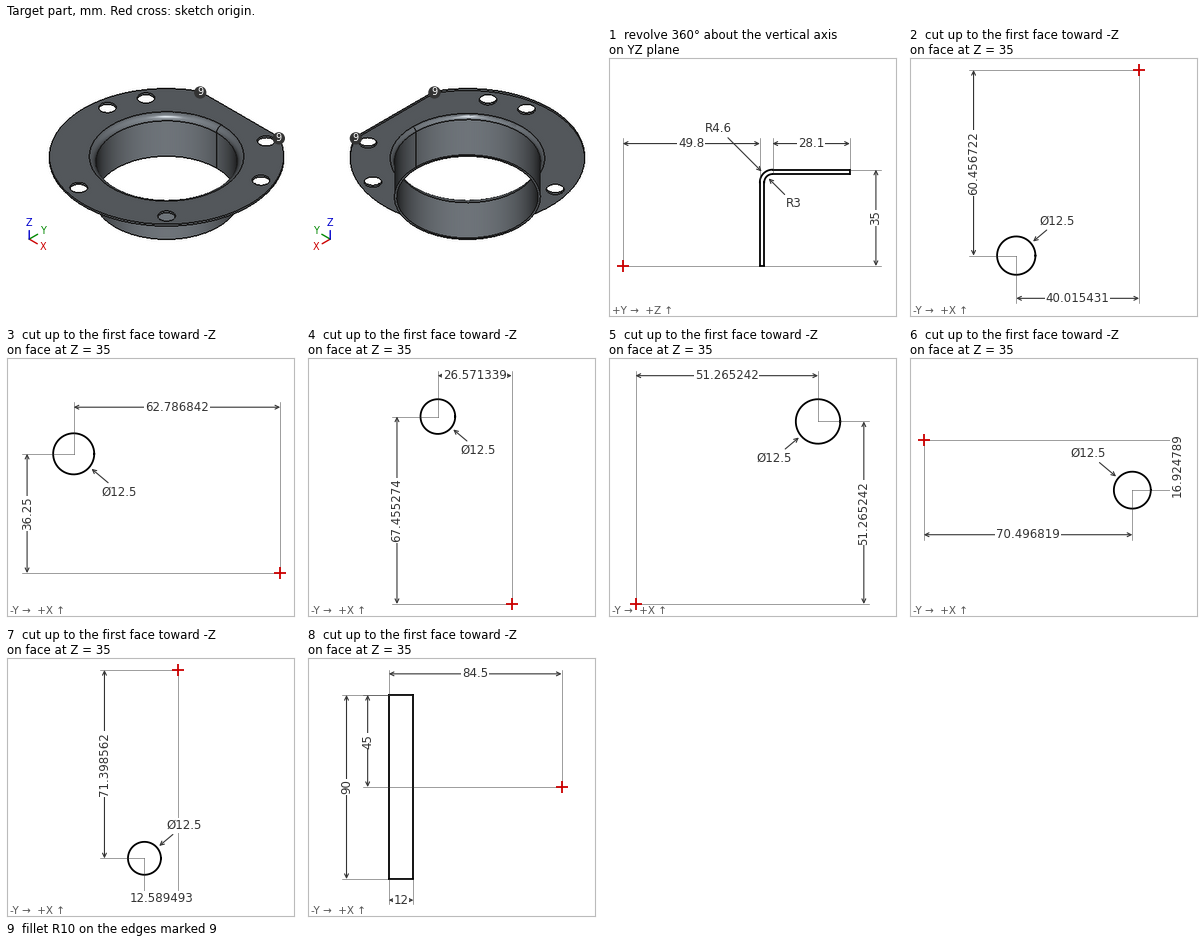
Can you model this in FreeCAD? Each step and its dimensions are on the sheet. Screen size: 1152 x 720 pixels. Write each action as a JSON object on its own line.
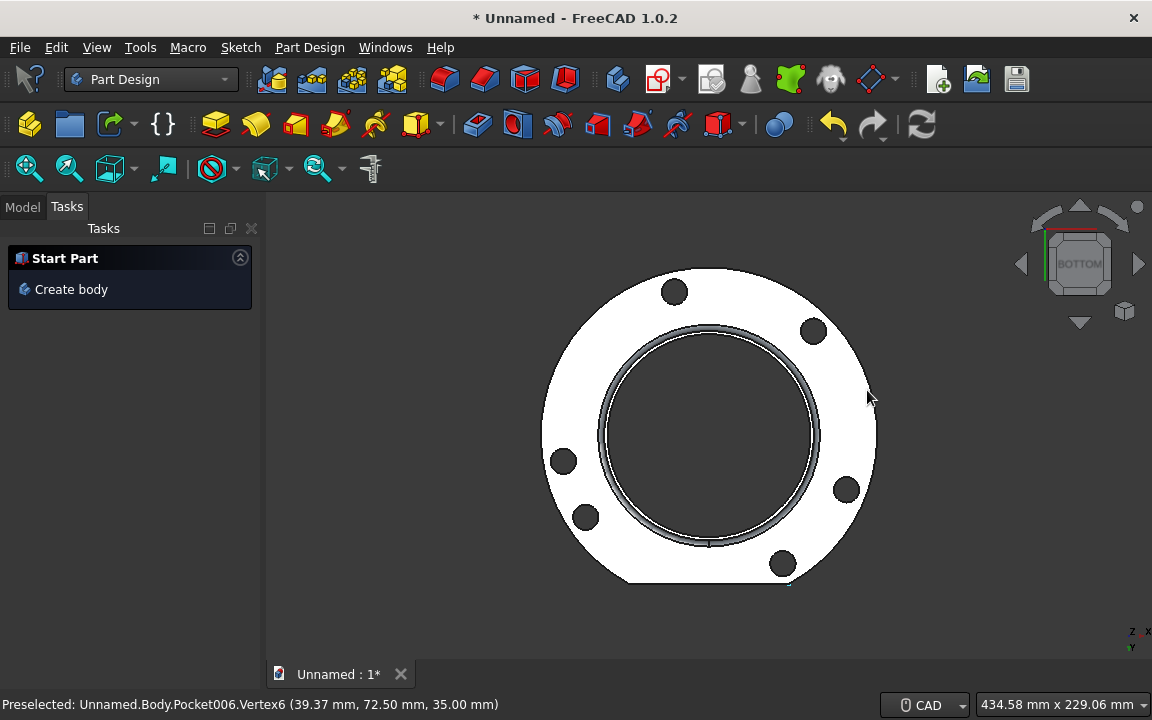
{"action": "scroll", "coordinate": [629, 583], "scroll_direction": "up", "scroll_amount": 13}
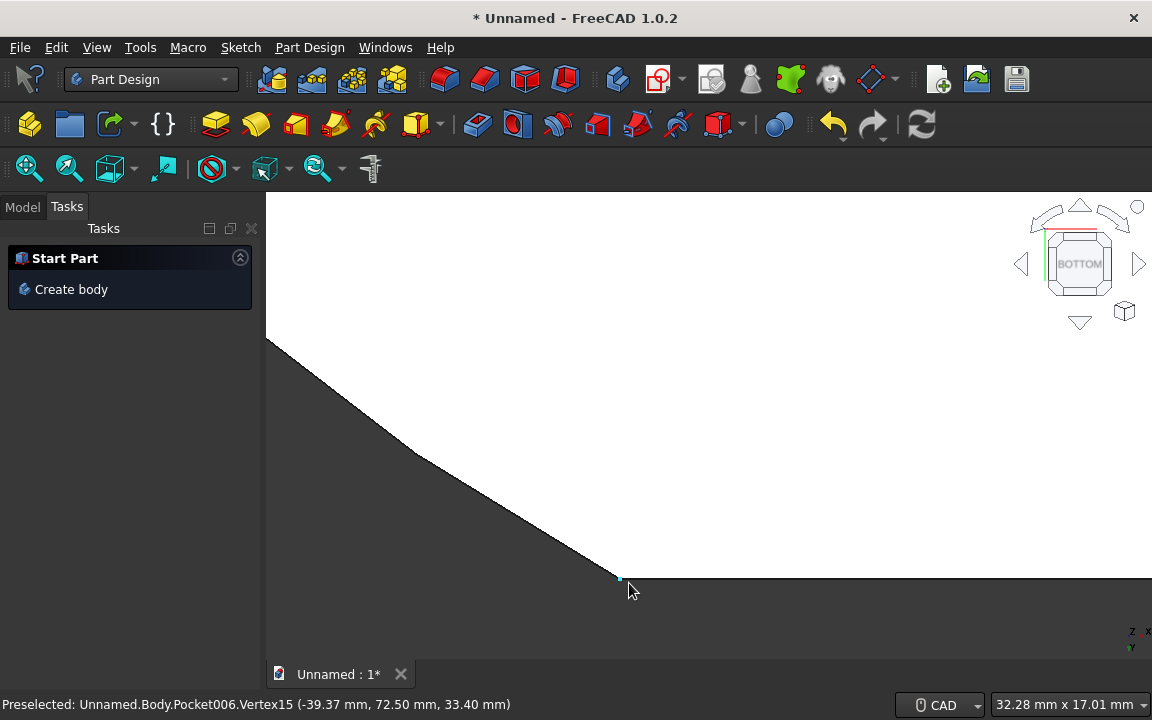
{"action": "key", "text": "v f"}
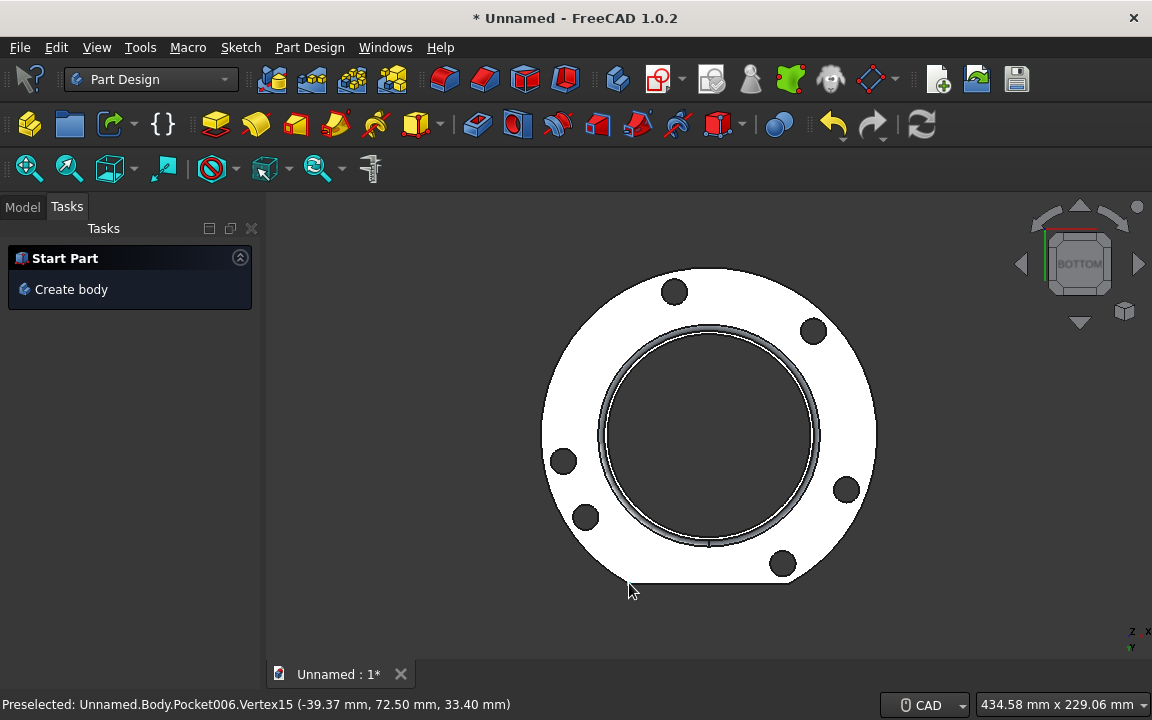
{"action": "key", "text": "4"}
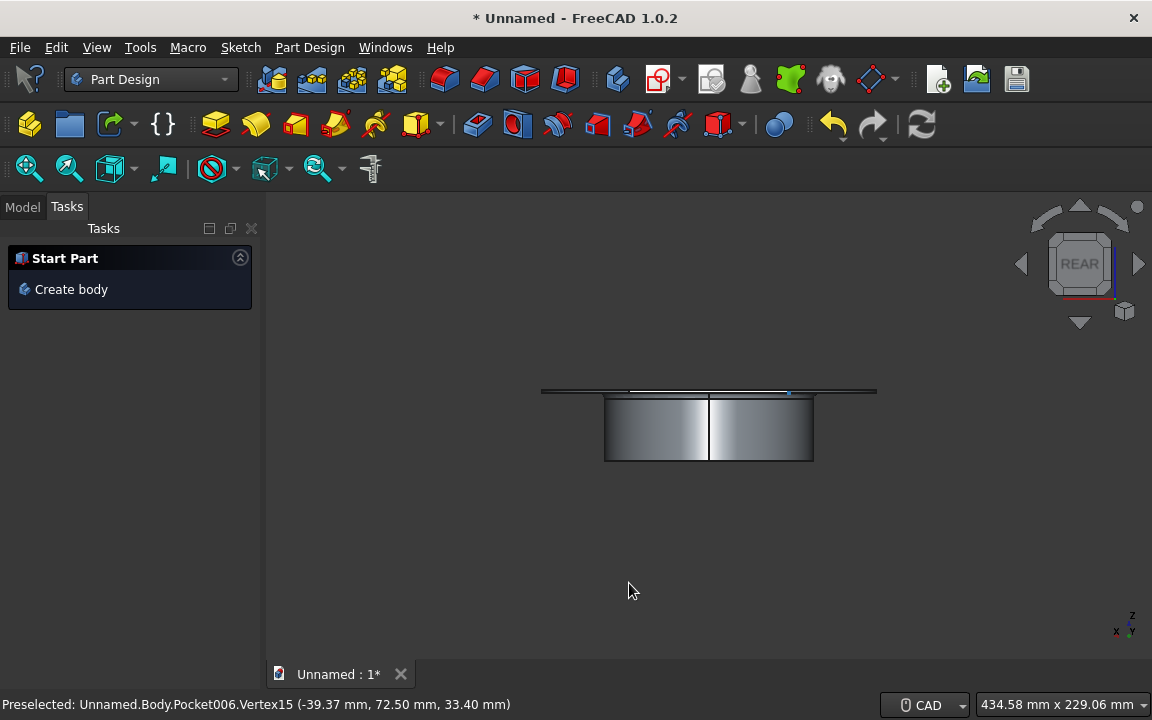
{"action": "key", "text": "v f"}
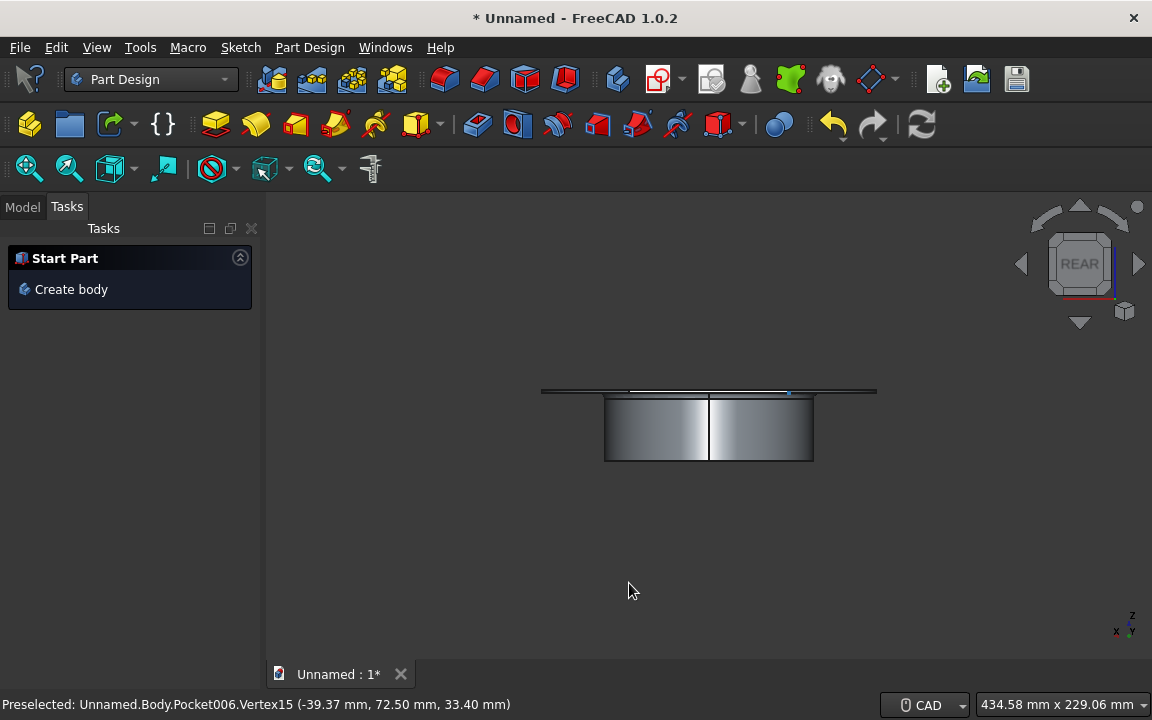
{"action": "scroll", "coordinate": [789, 390], "scroll_direction": "up", "scroll_amount": 13}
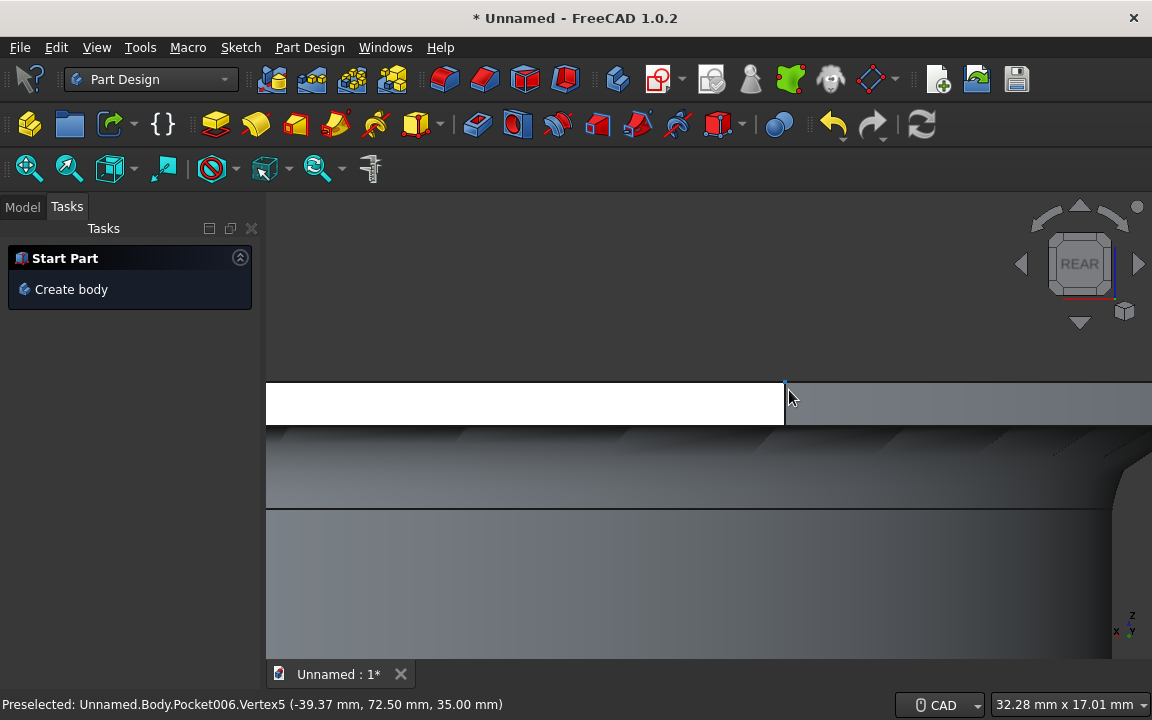
{"action": "left_click", "coordinate": [785, 403]}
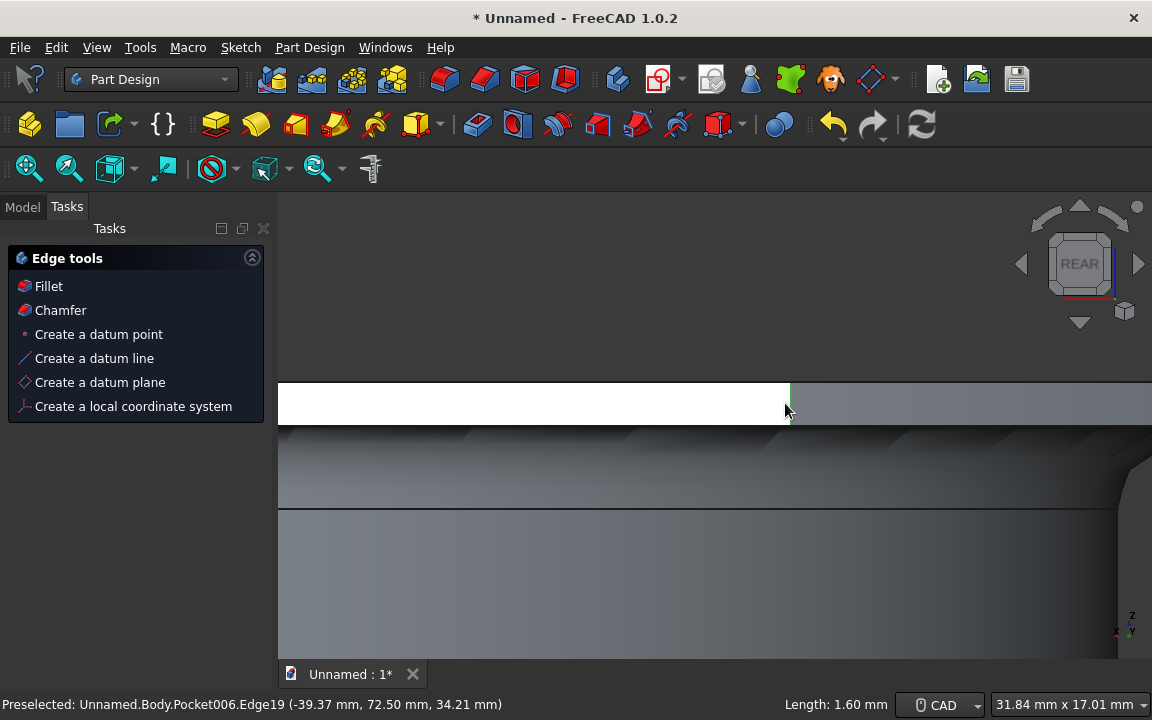
{"action": "key", "text": "v f"}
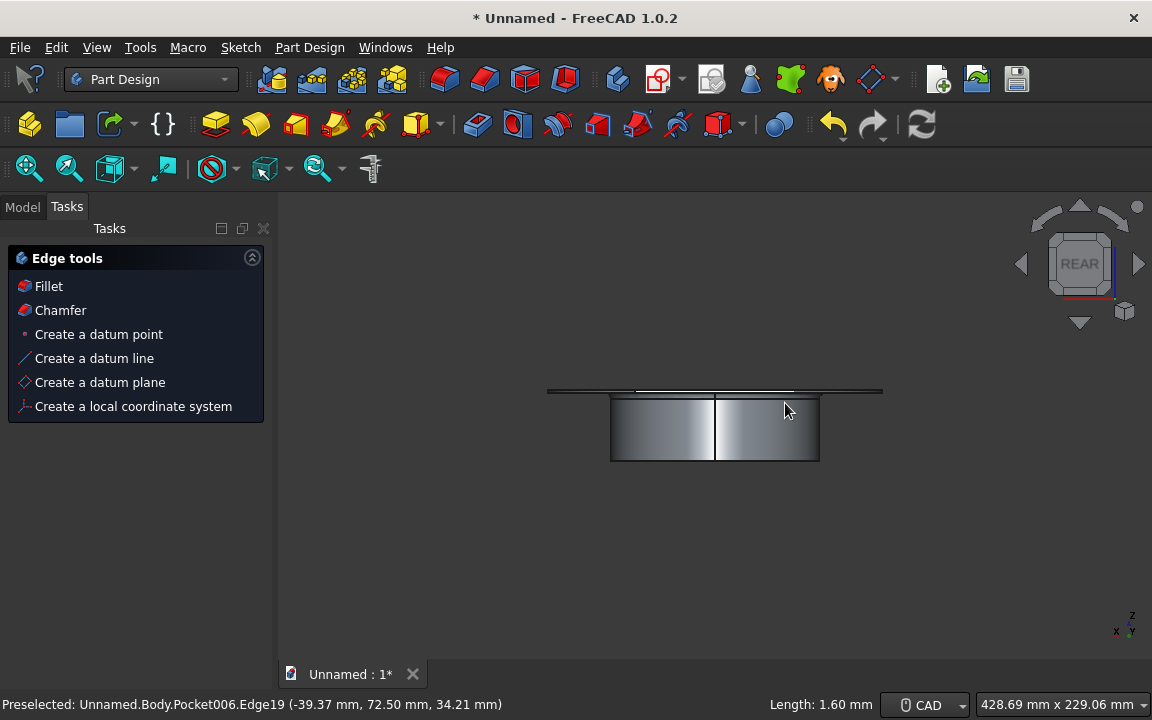
{"action": "key", "text": "6"}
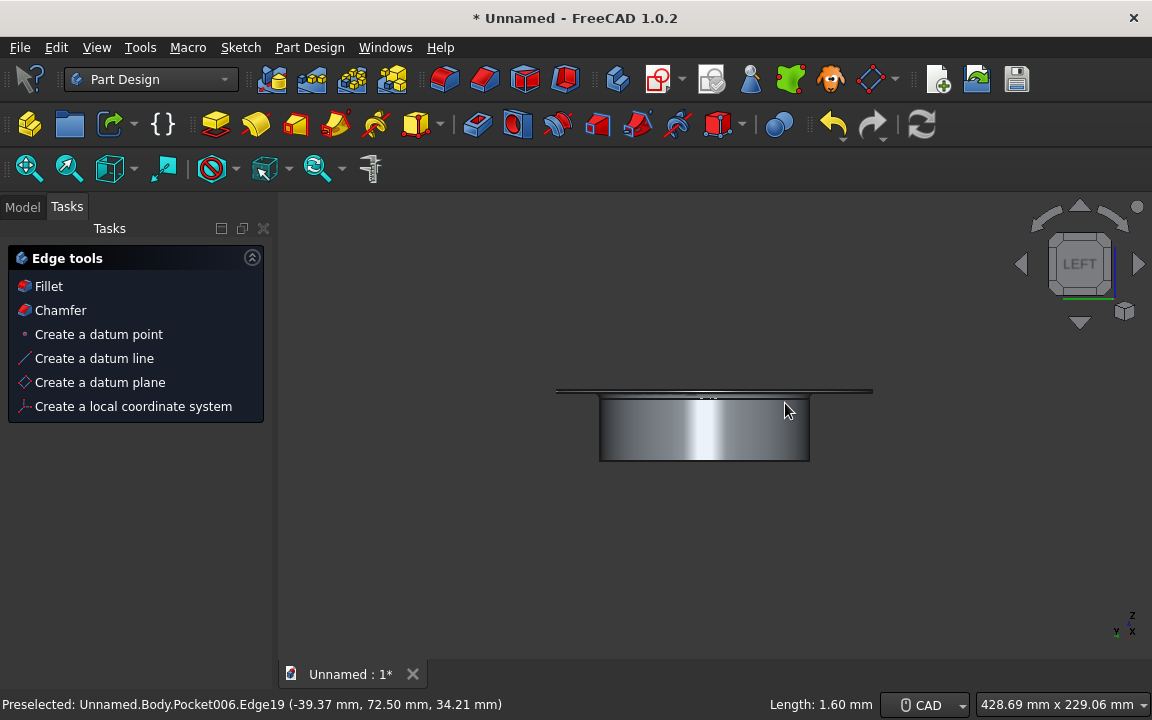
{"action": "key", "text": "v f"}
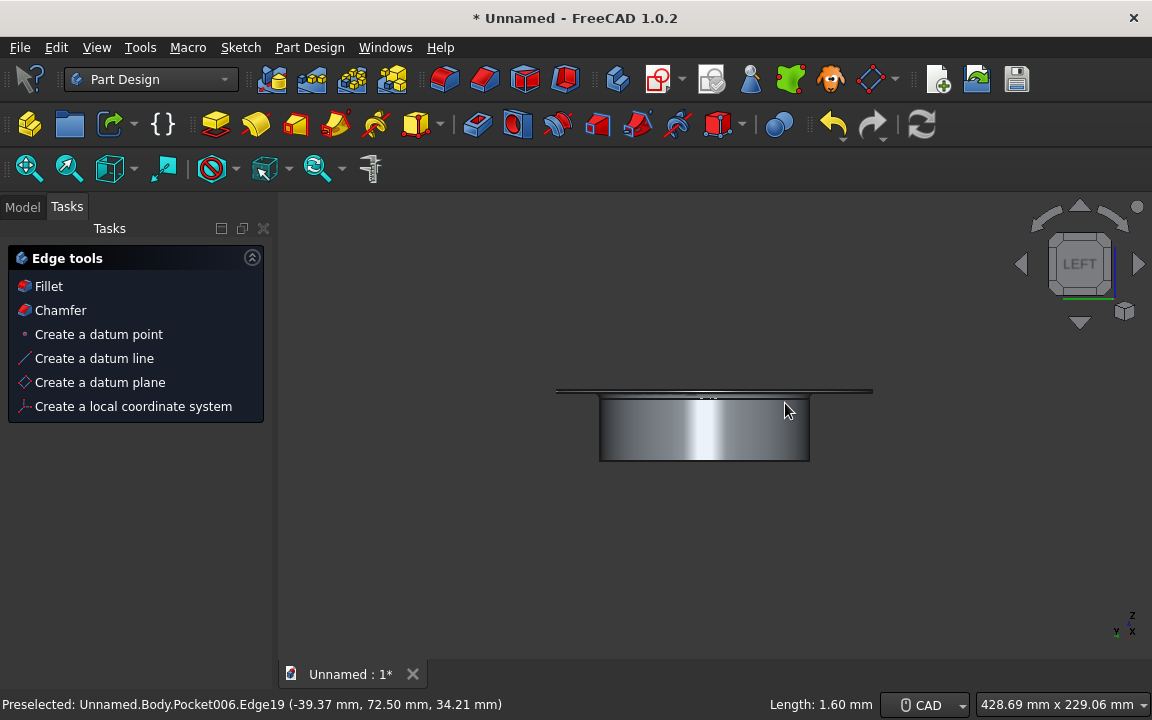
{"action": "scroll", "coordinate": [557, 390], "scroll_direction": "up", "scroll_amount": 13}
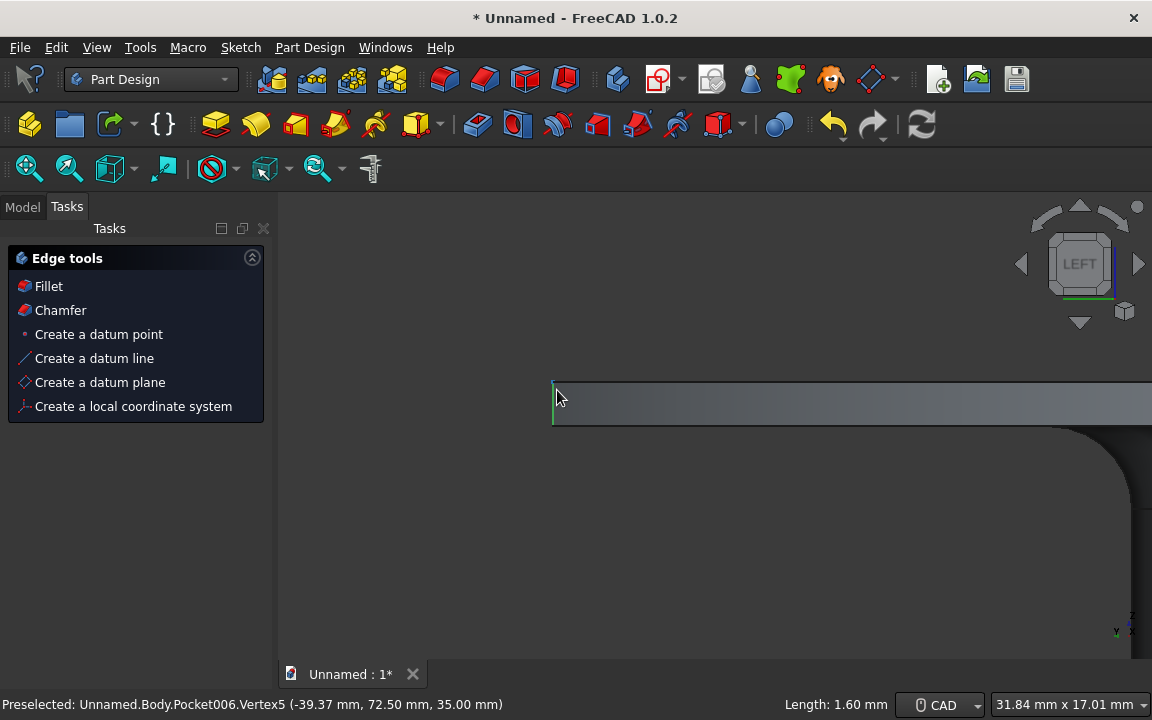
{"action": "key", "text": "v f"}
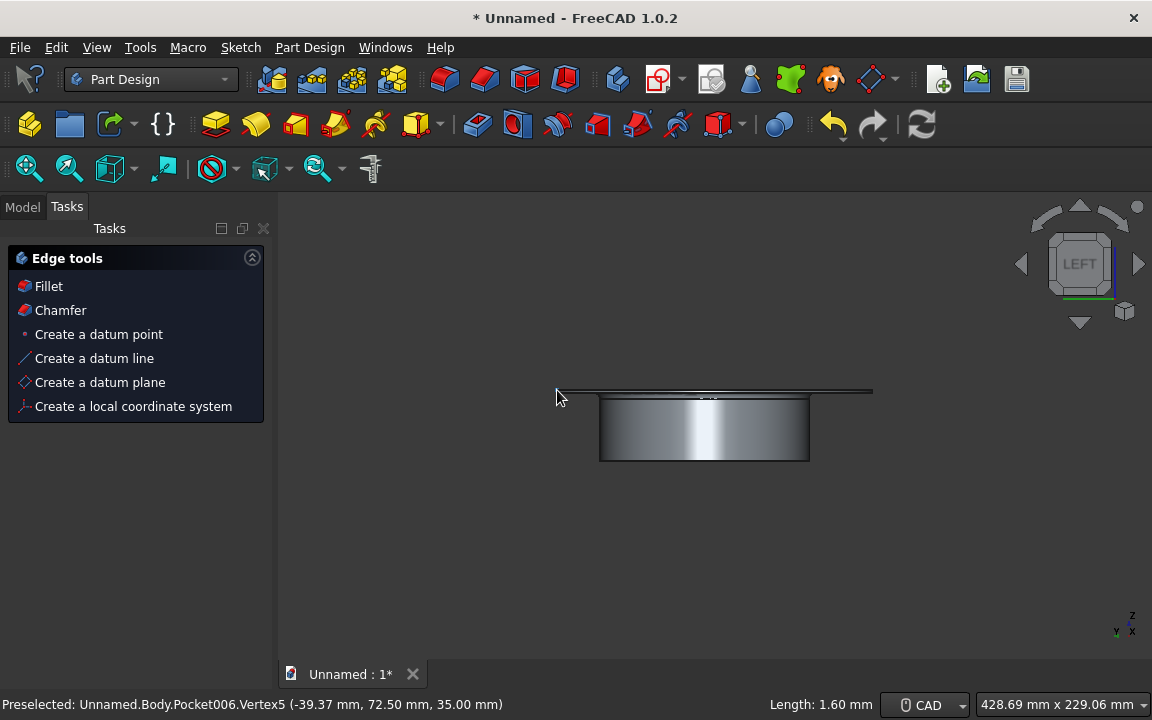
{"action": "key", "text": "v 3"}